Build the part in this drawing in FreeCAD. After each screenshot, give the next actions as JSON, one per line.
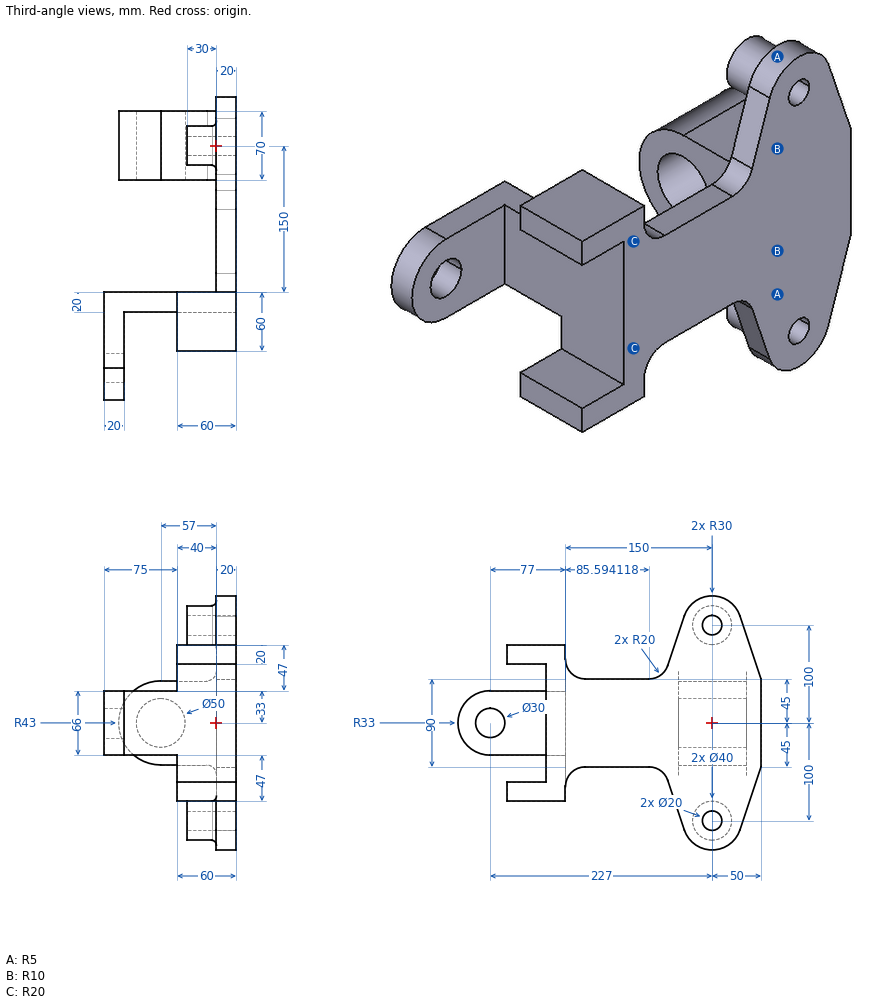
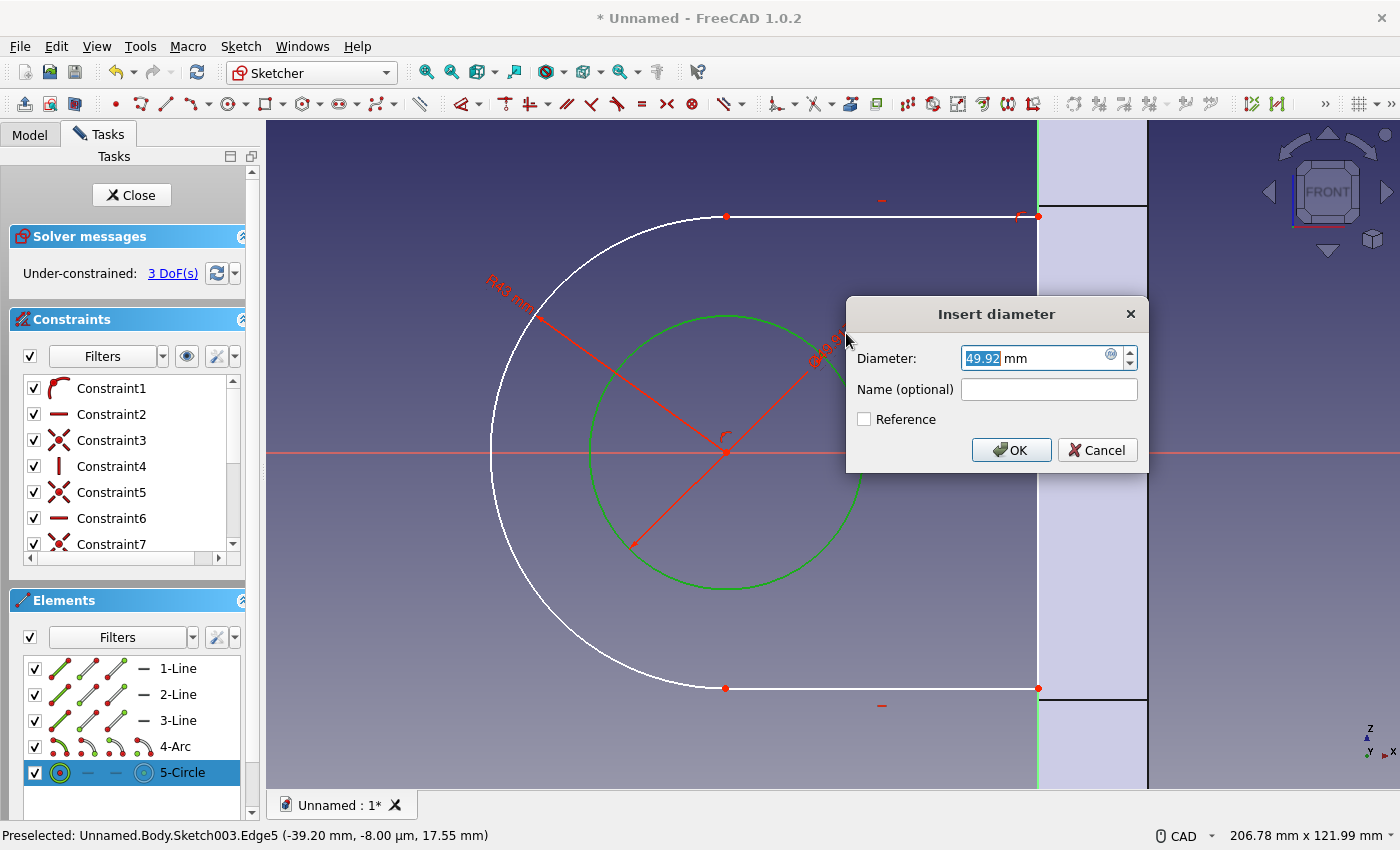
{"action": "type", "text": "50"}
{"action": "key", "text": "Return"}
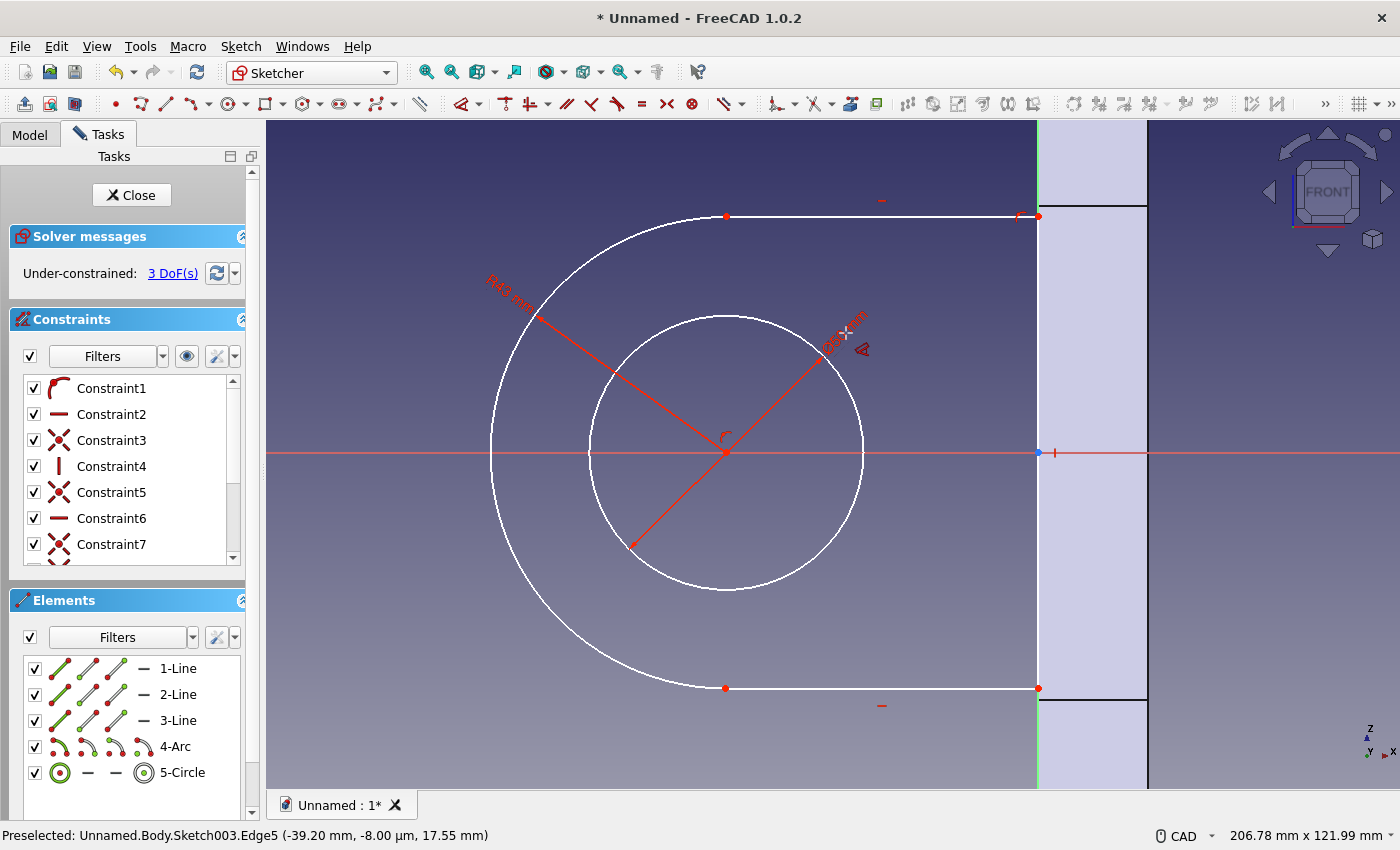
{"action": "left_click", "coordinate": [820, 217]}
{"action": "left_click", "coordinate": [882, 183]}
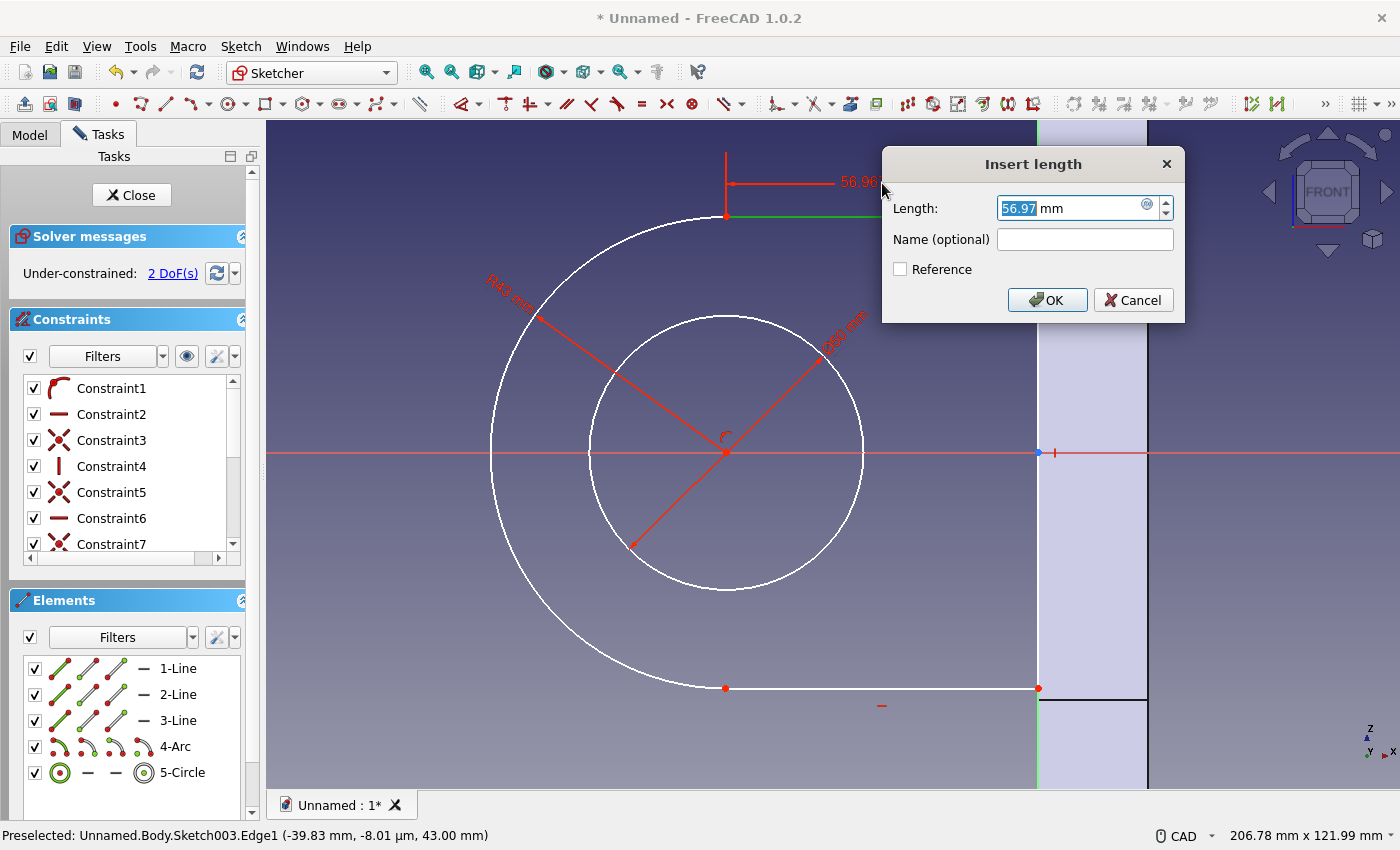
{"action": "type", "text": "57"}
{"action": "key", "text": "Return"}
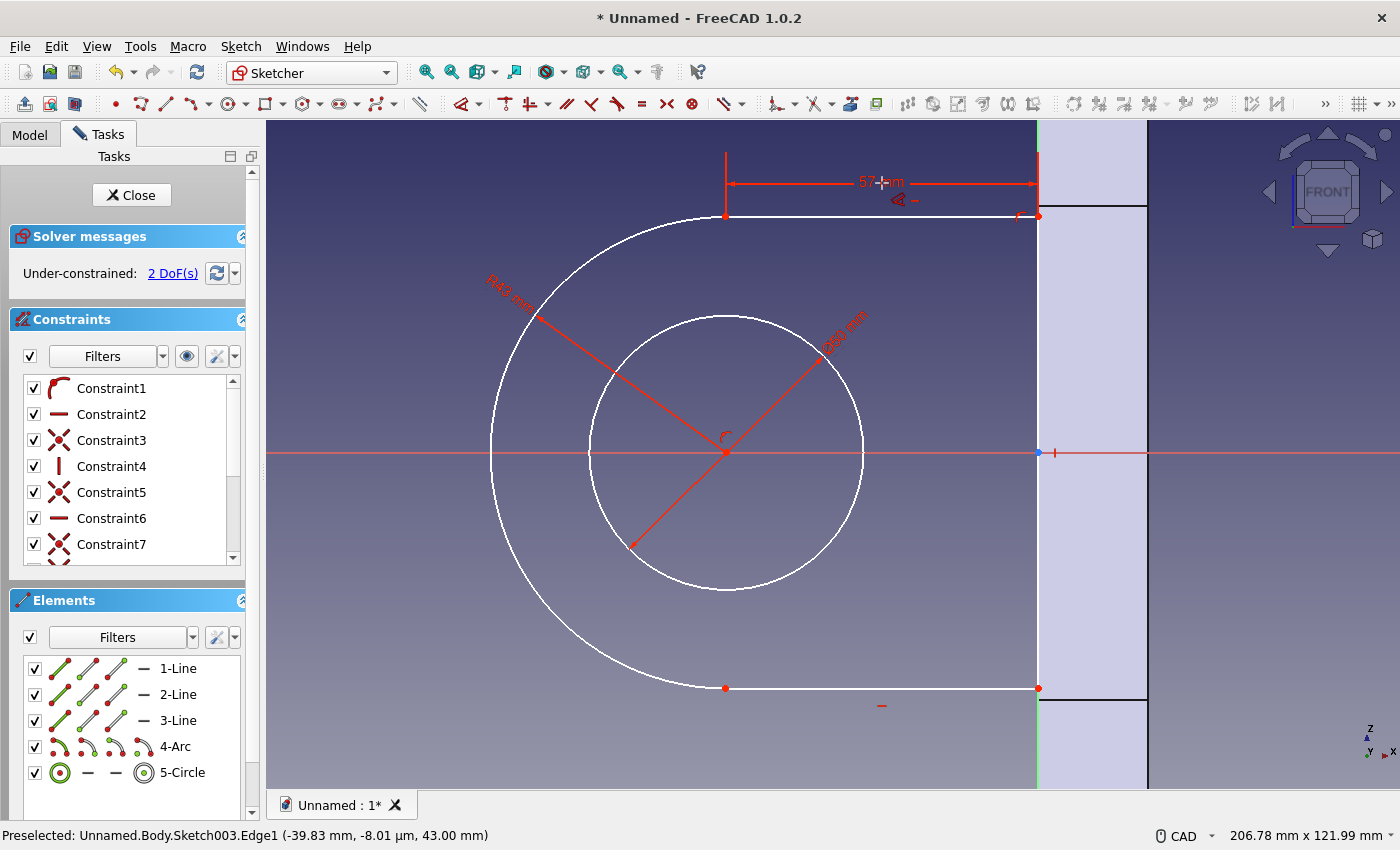
{"action": "left_click", "coordinate": [945, 689]}
{"action": "left_click", "coordinate": [882, 723]}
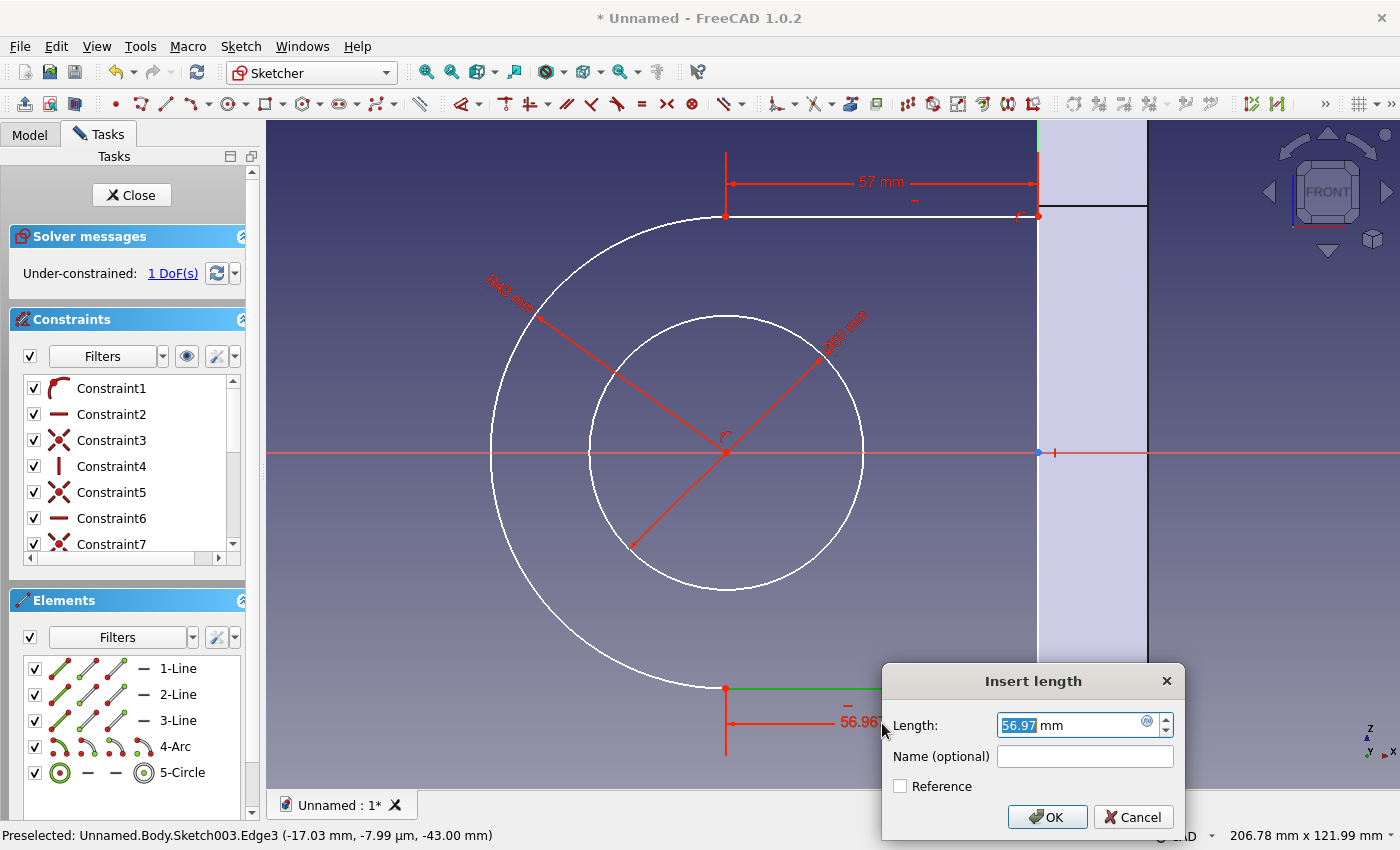
{"action": "type", "text": "57"}
{"action": "key", "text": "Return"}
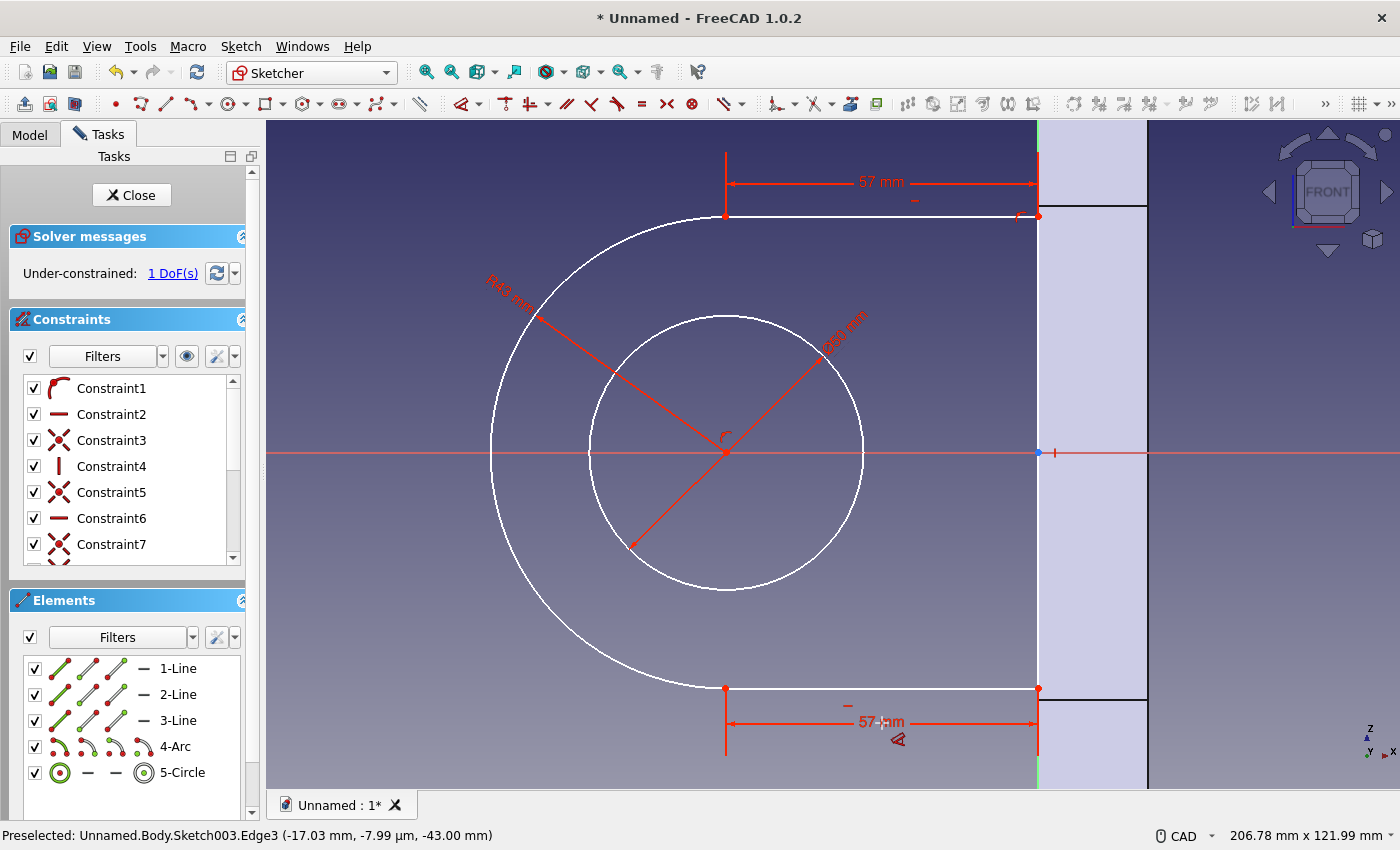
{"action": "left_click", "coordinate": [726, 453]}
{"action": "left_click", "coordinate": [882, 487]}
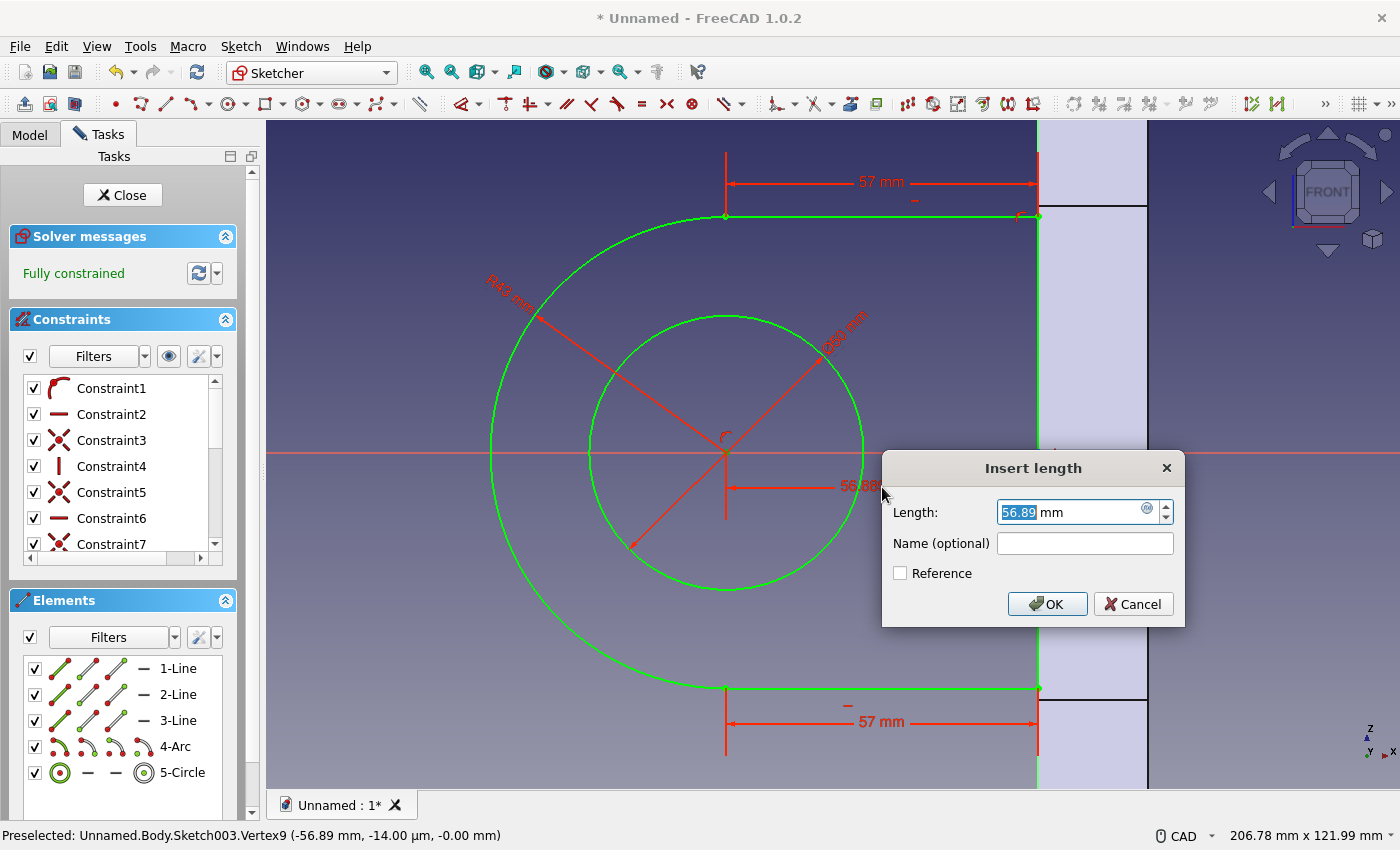
{"action": "type", "text": "57"}
{"action": "key", "text": "Return"}
{"action": "key", "text": "Escape"}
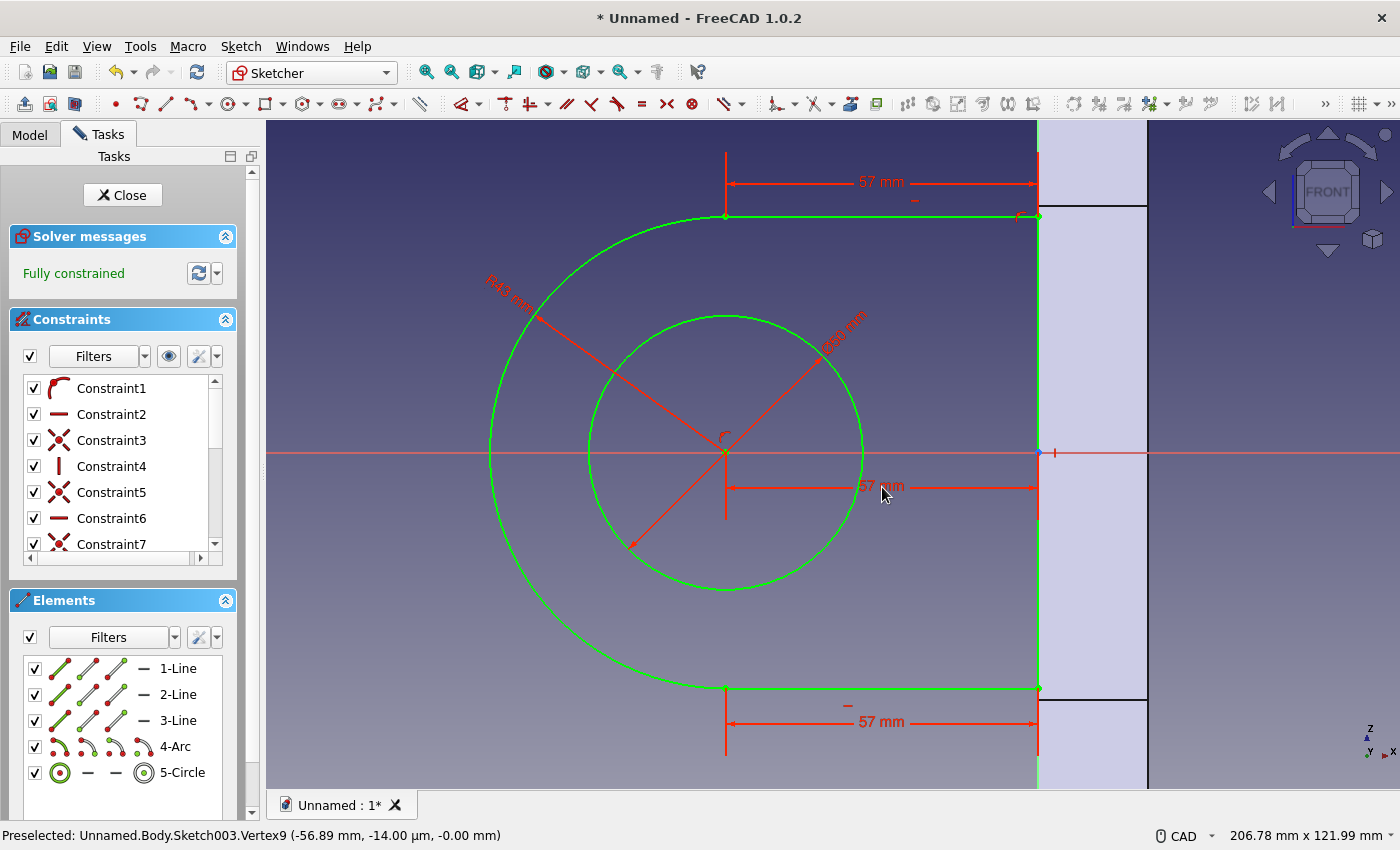
{"action": "left_click", "coordinate": [123, 195]}